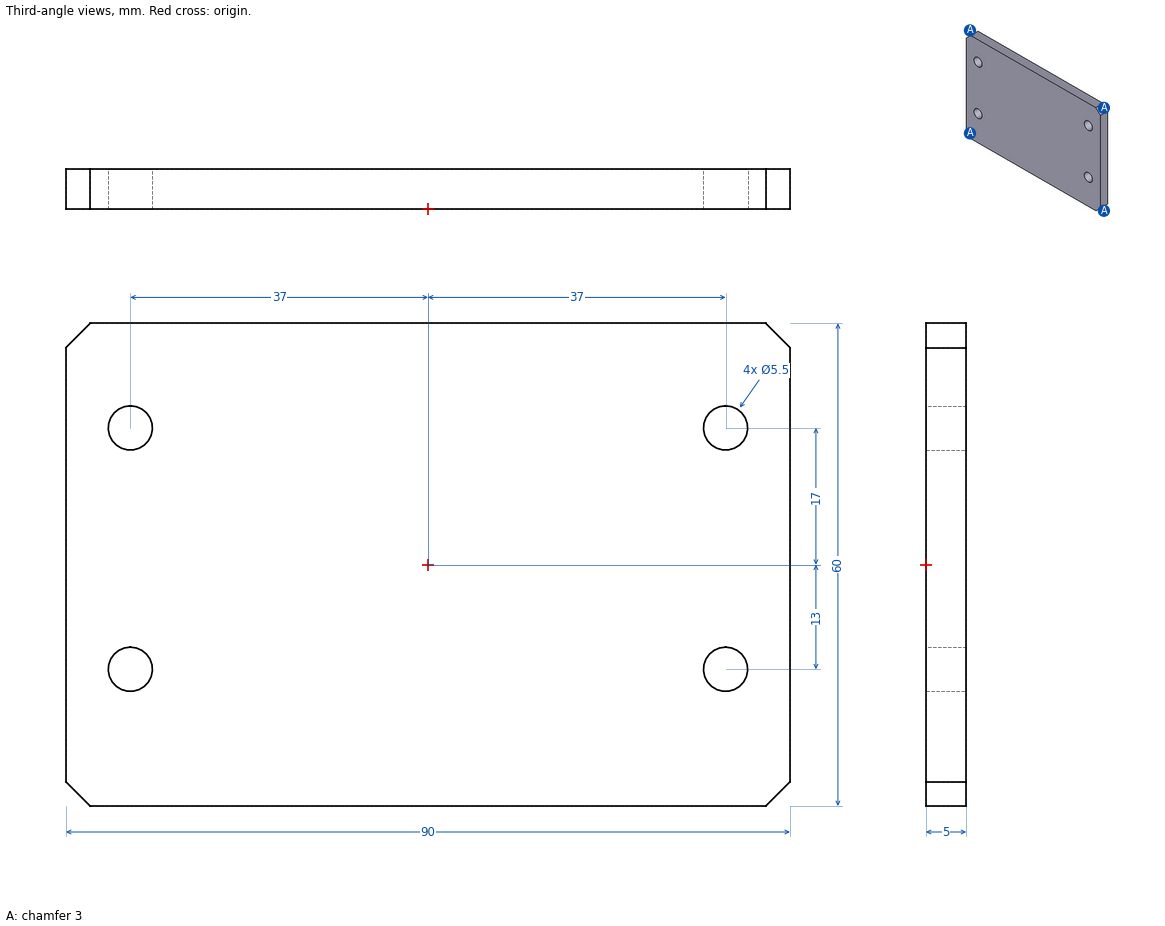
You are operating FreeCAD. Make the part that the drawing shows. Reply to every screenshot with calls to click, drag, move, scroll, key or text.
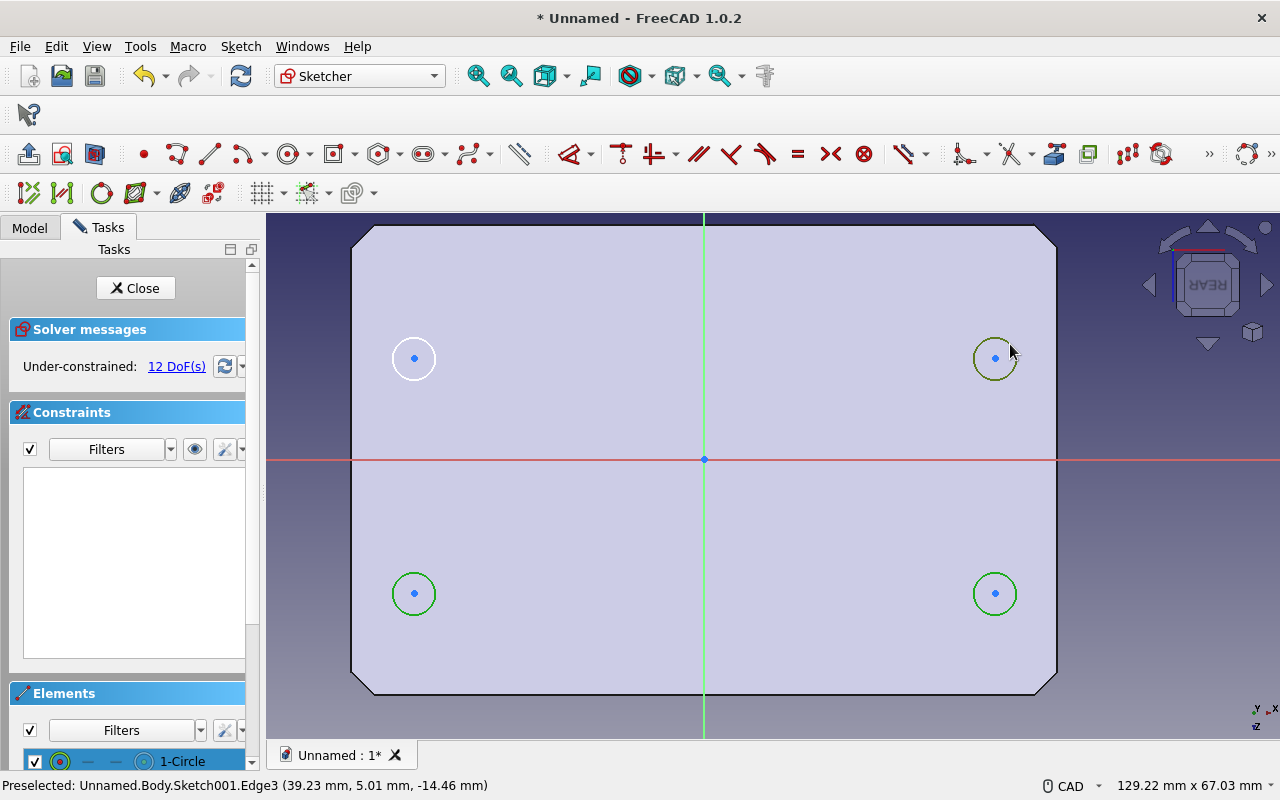
click(429, 344)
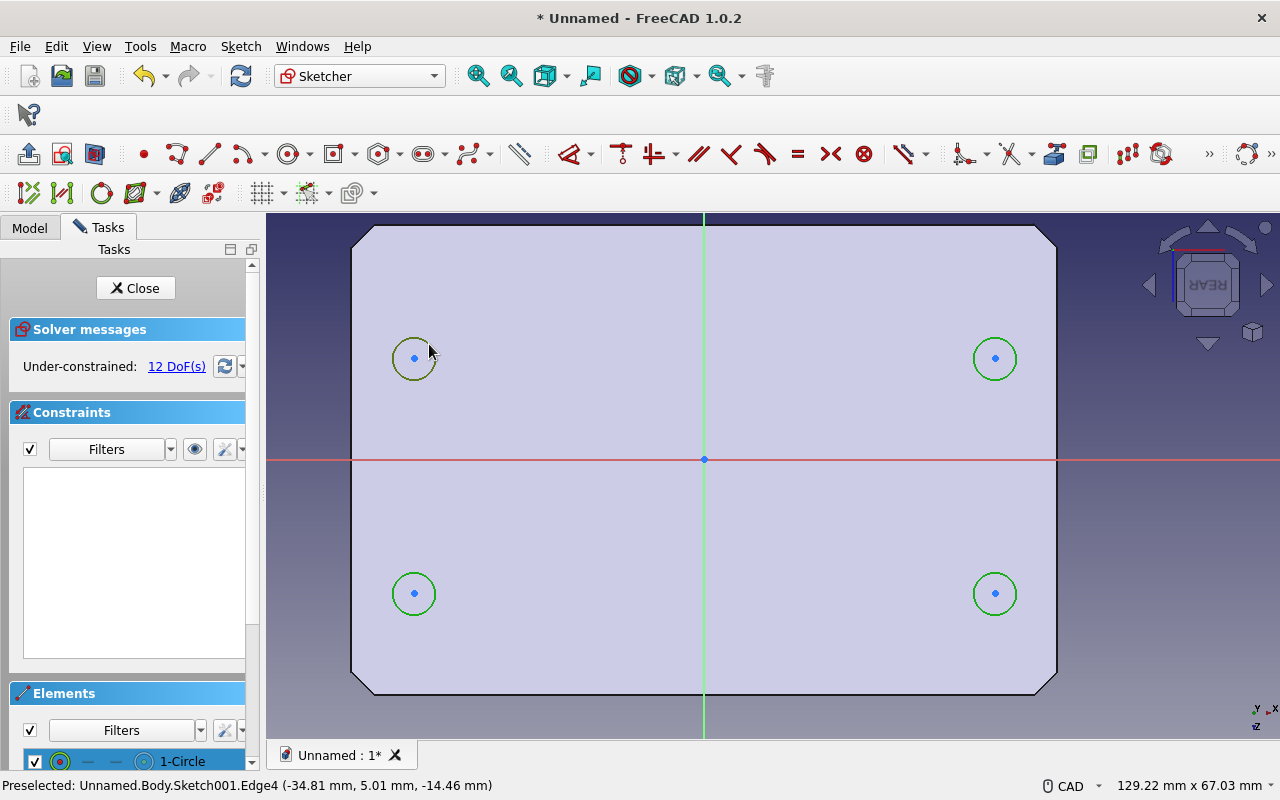
click(798, 154)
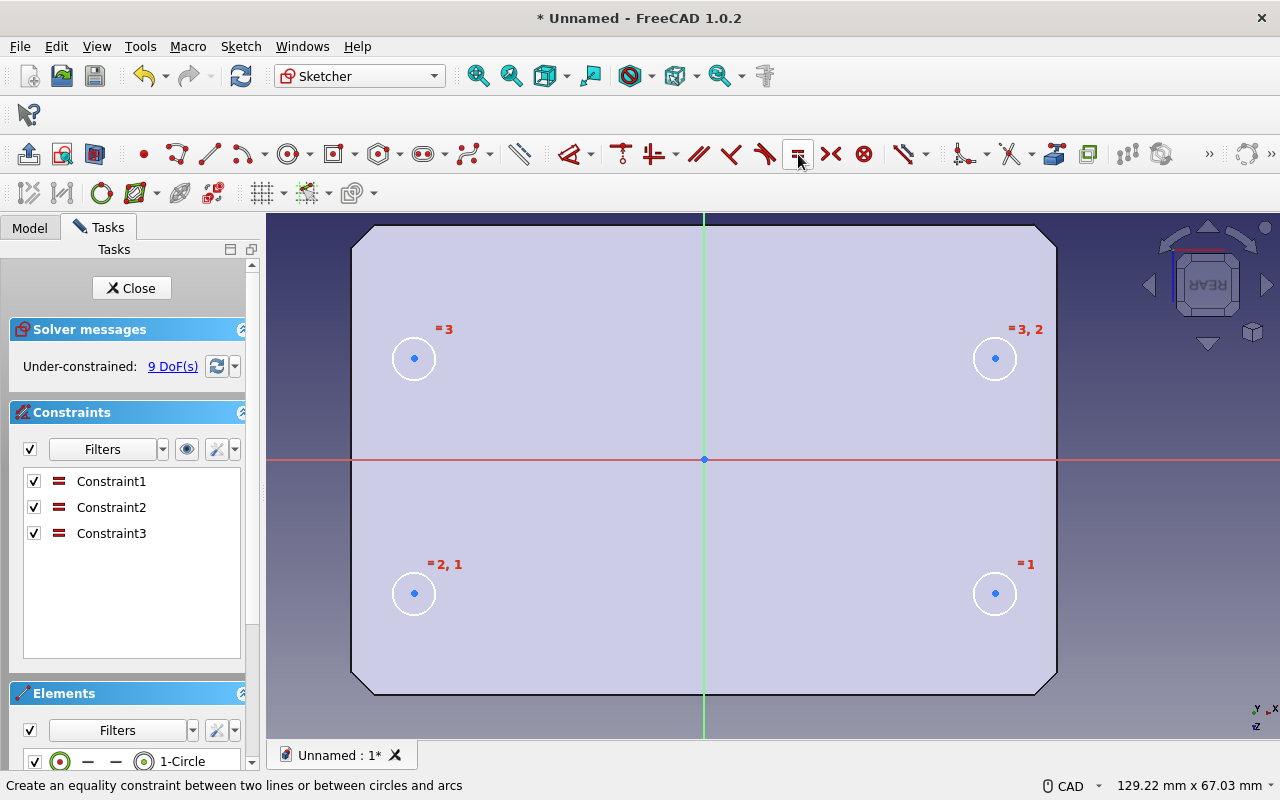
click(995, 594)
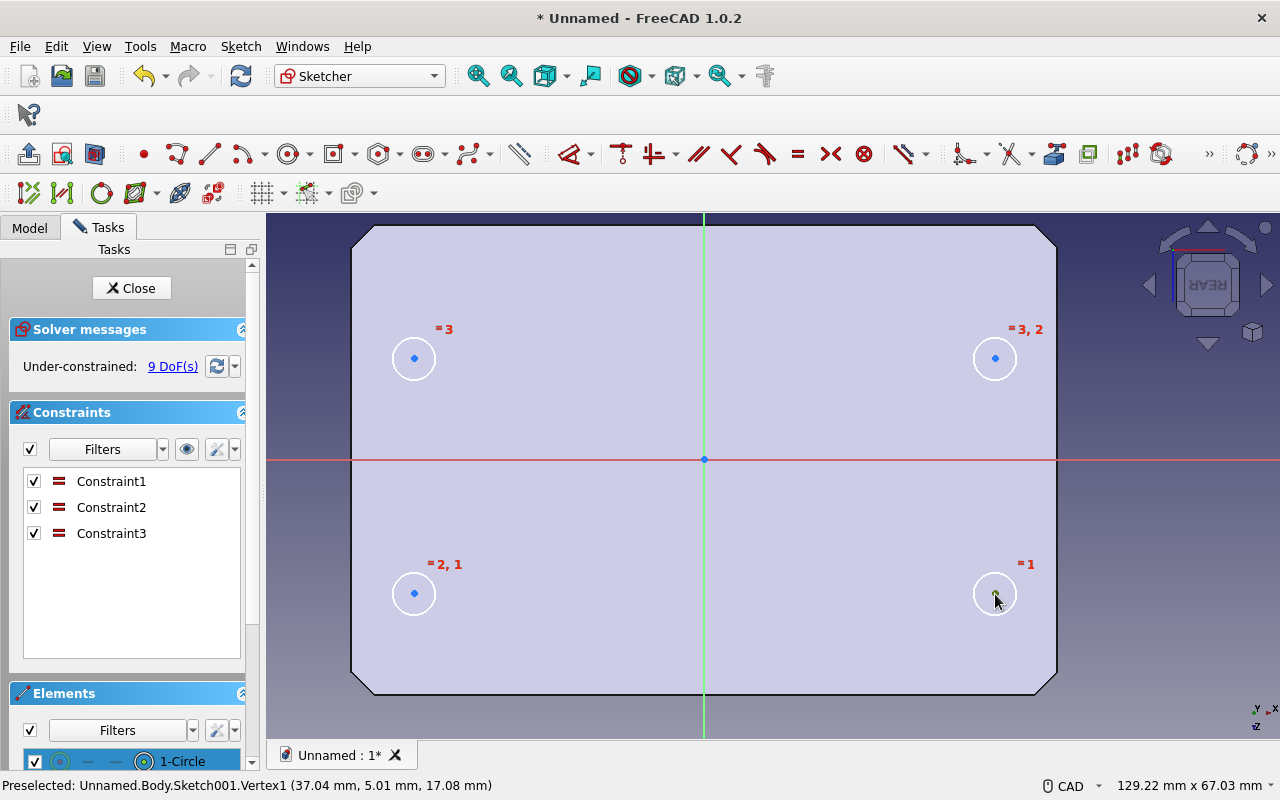
click(414, 594)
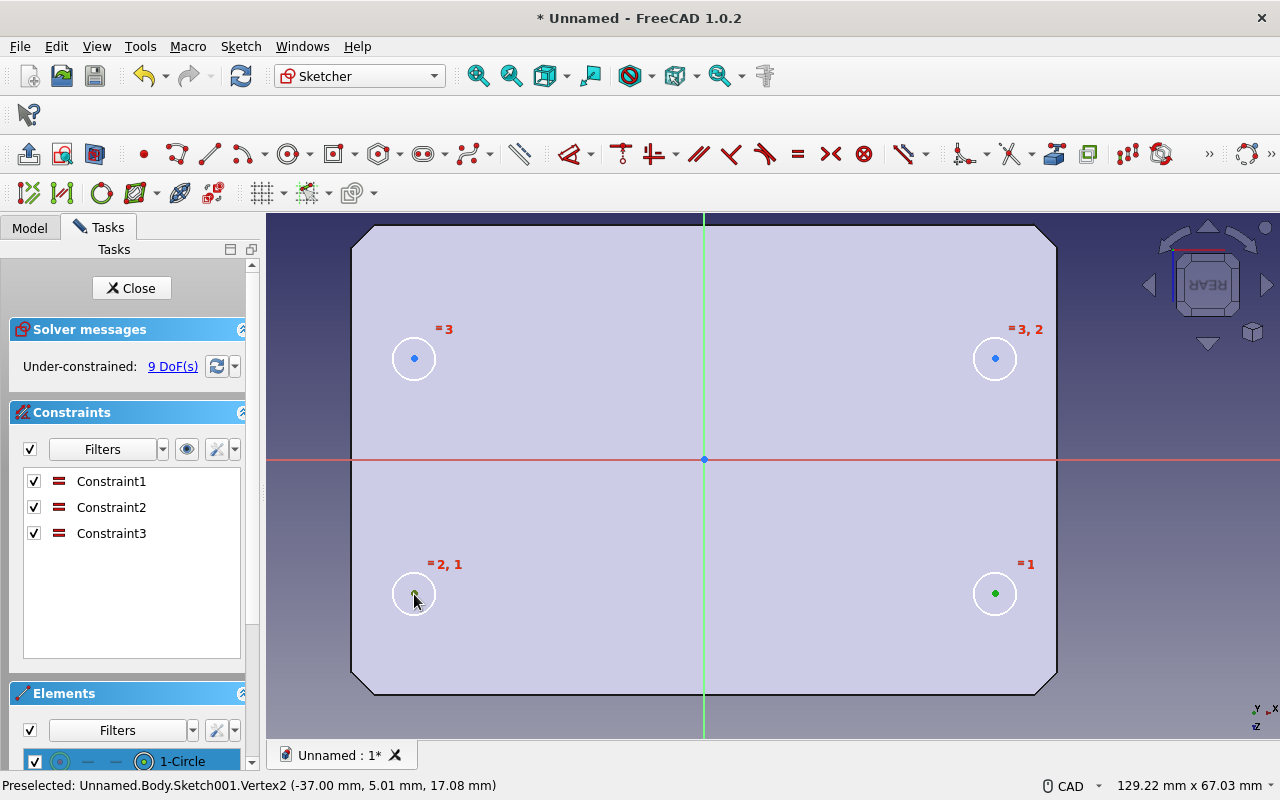
click(676, 154)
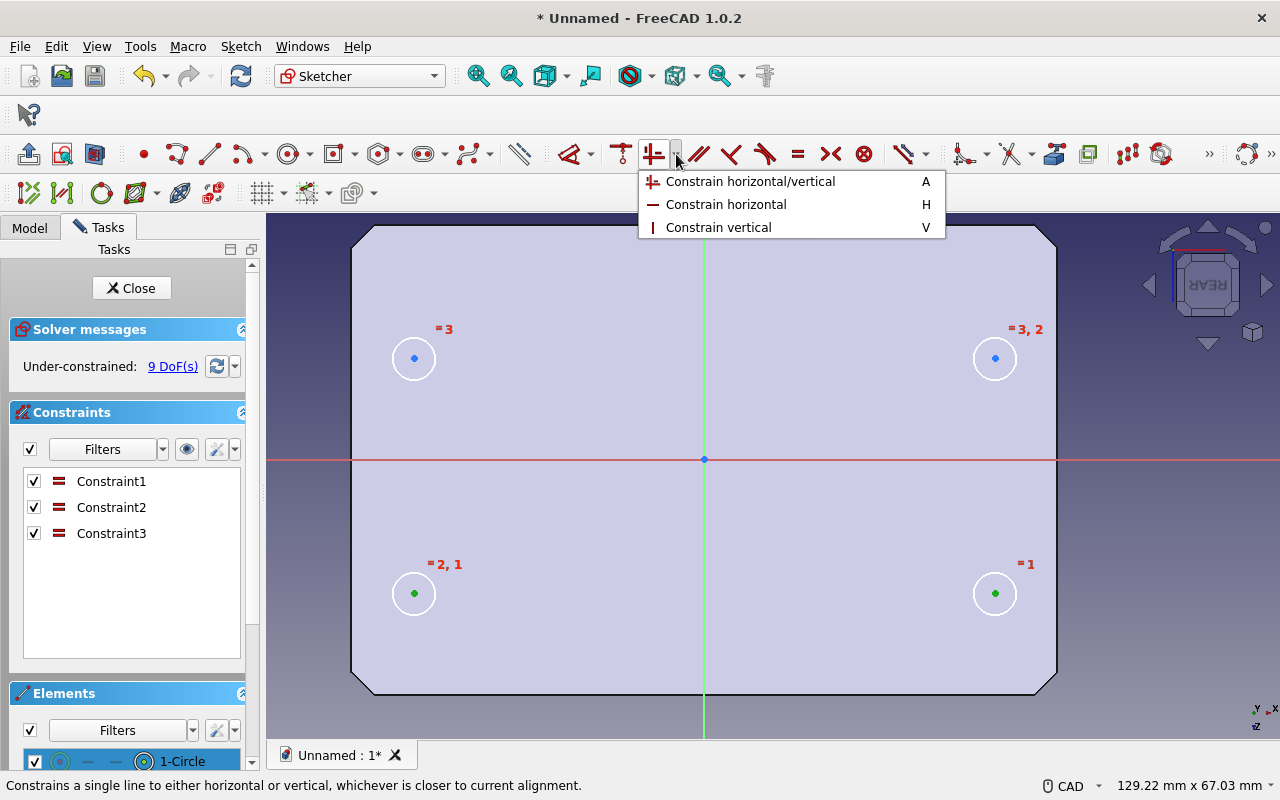
click(792, 204)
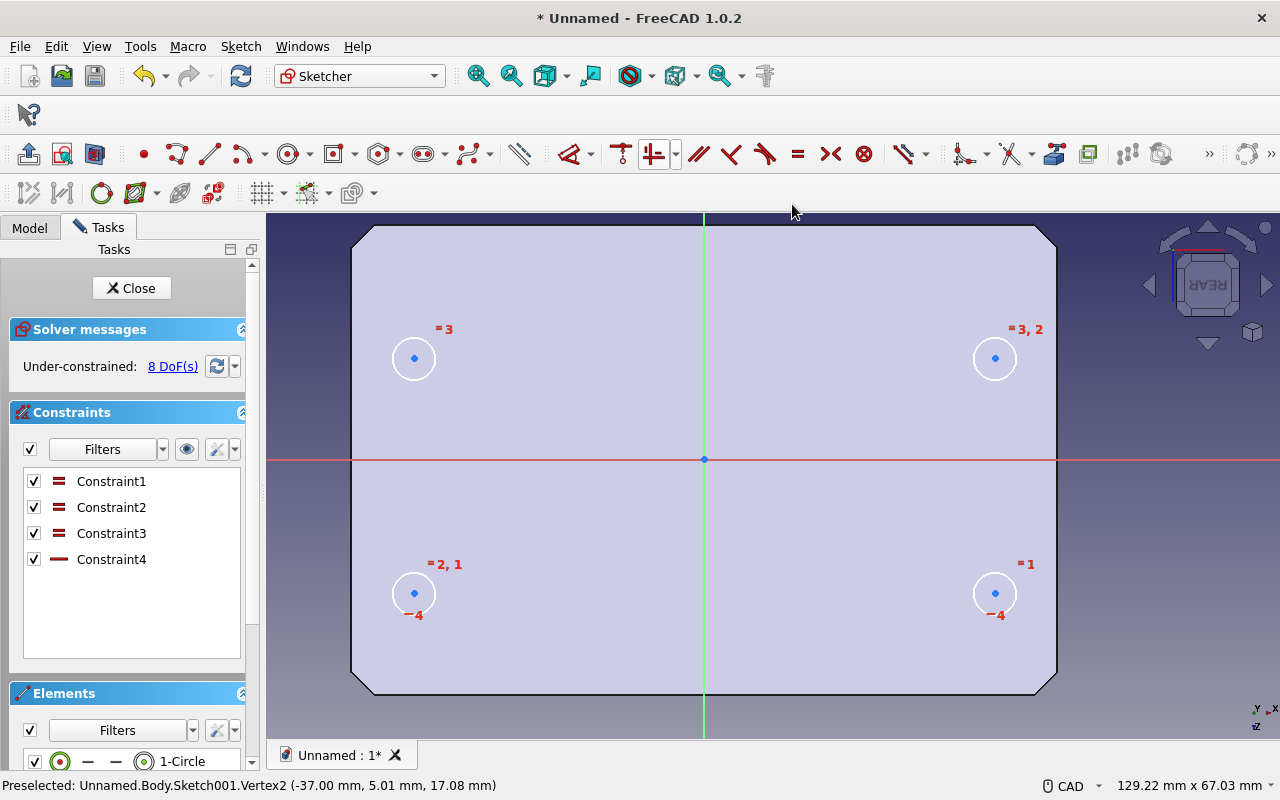
click(995, 594)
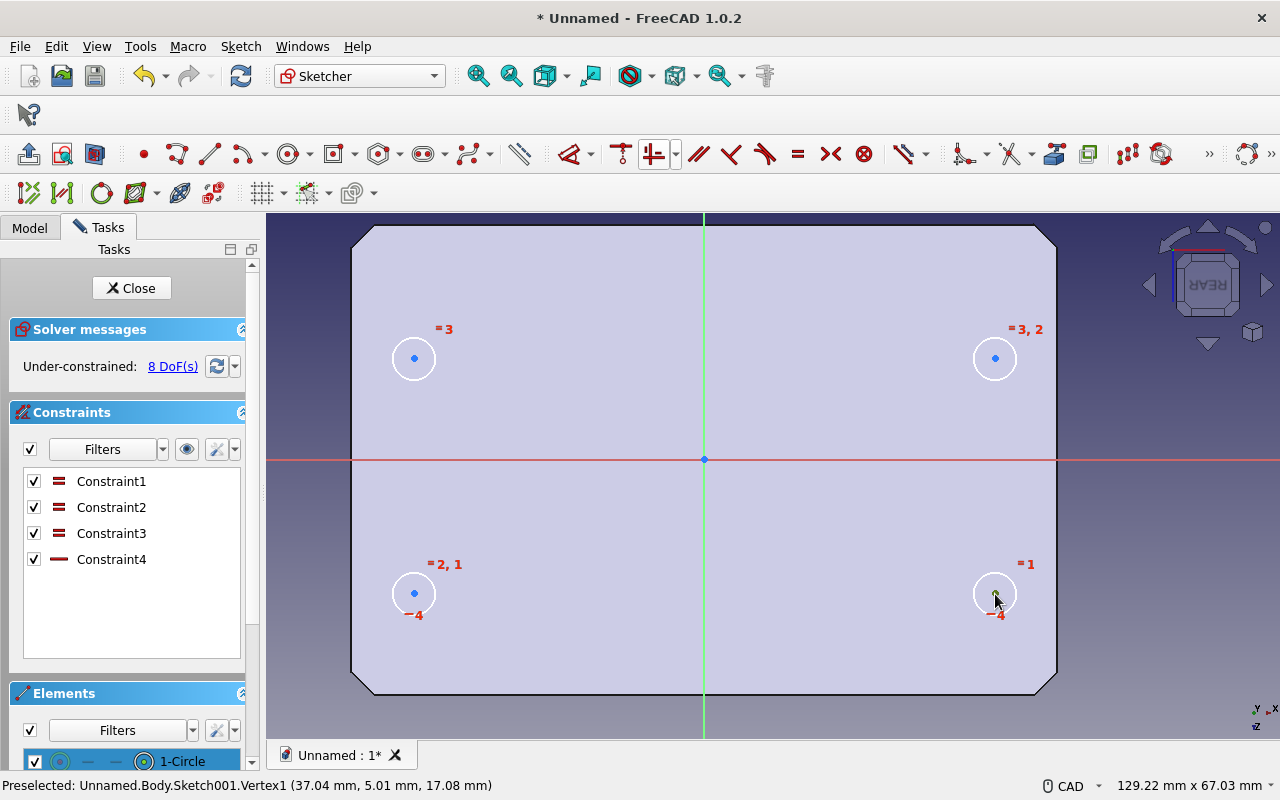
click(995, 359)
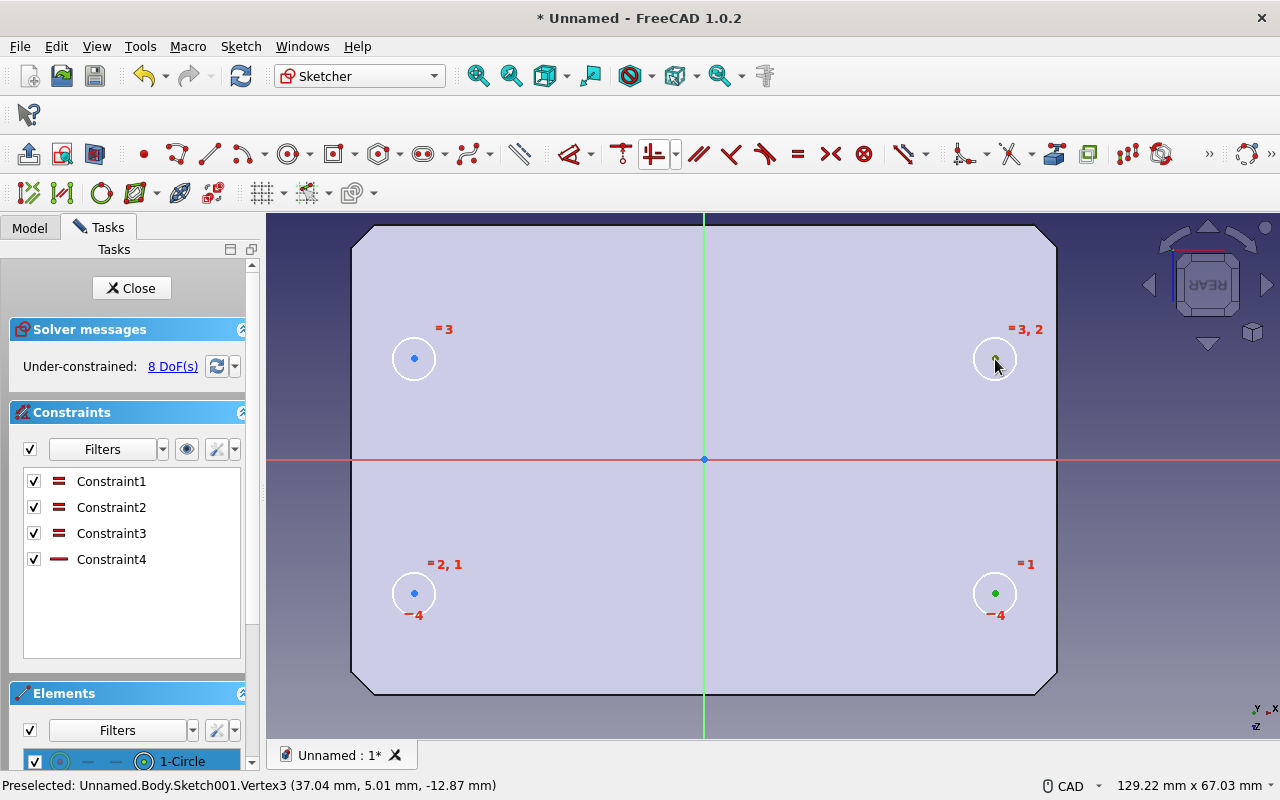
click(676, 154)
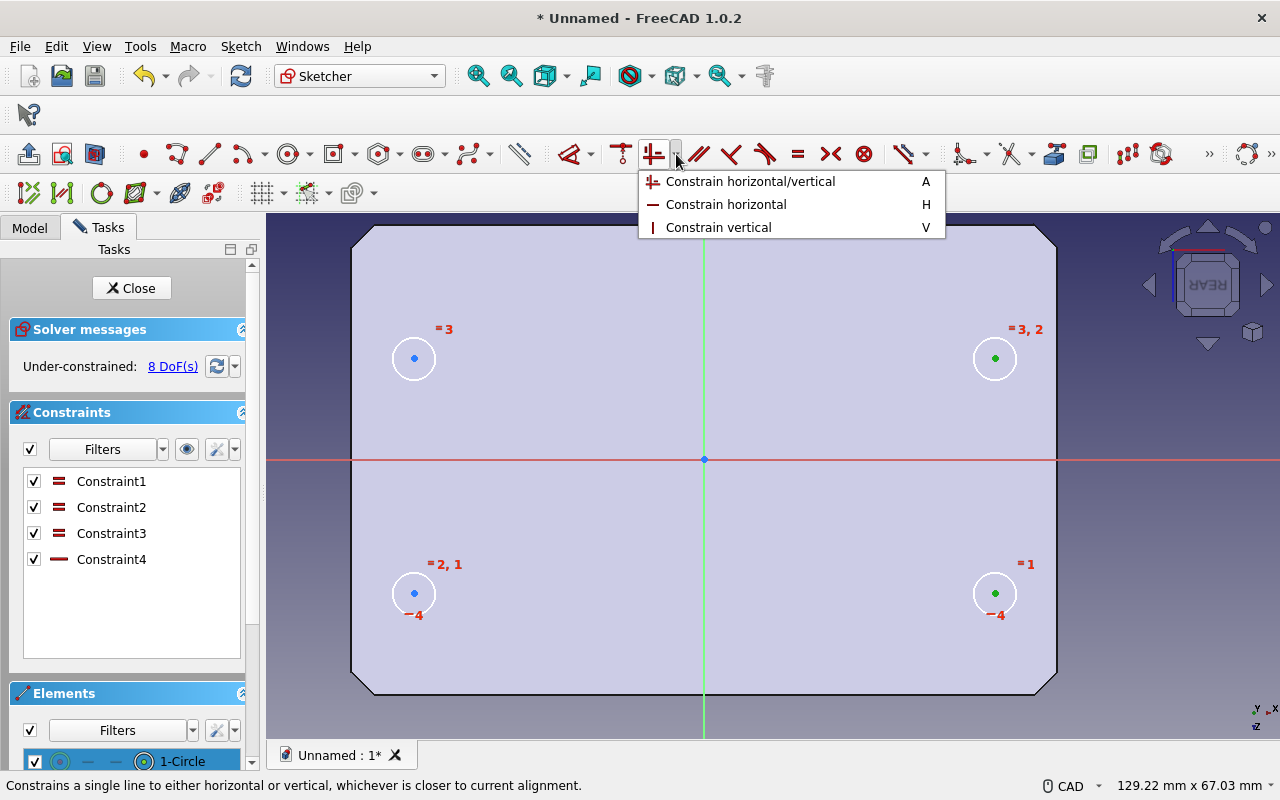
click(792, 228)